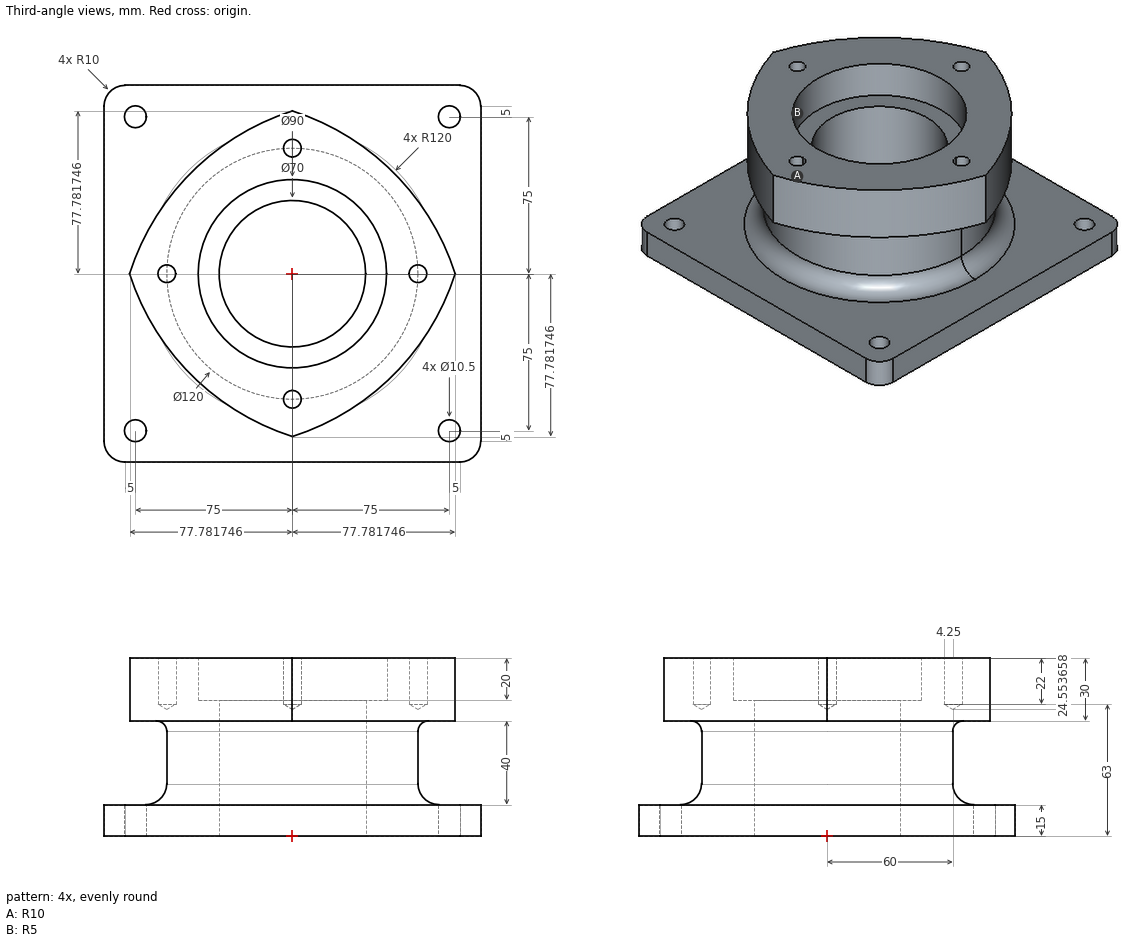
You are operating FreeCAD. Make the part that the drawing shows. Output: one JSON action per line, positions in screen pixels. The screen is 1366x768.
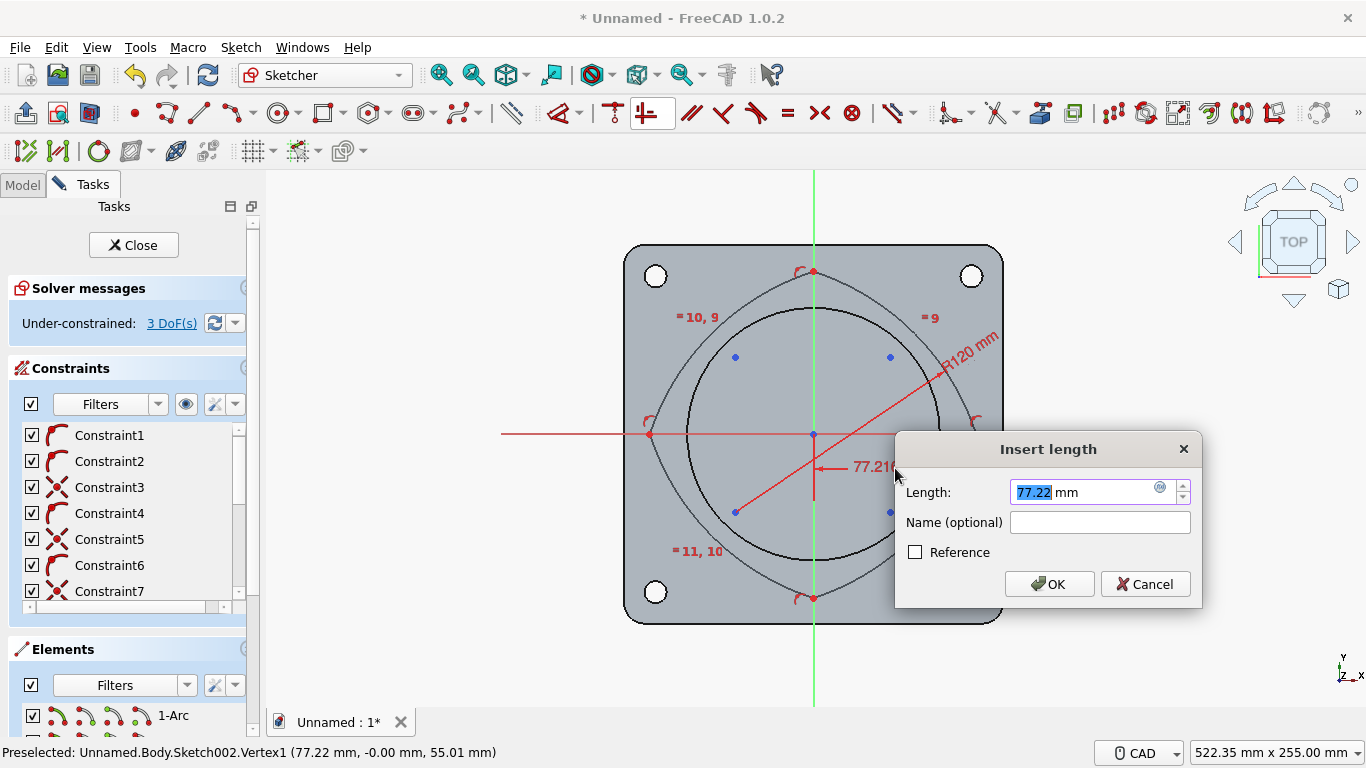
{"action": "type", "text": "77.781746"}
{"action": "key", "text": "Return"}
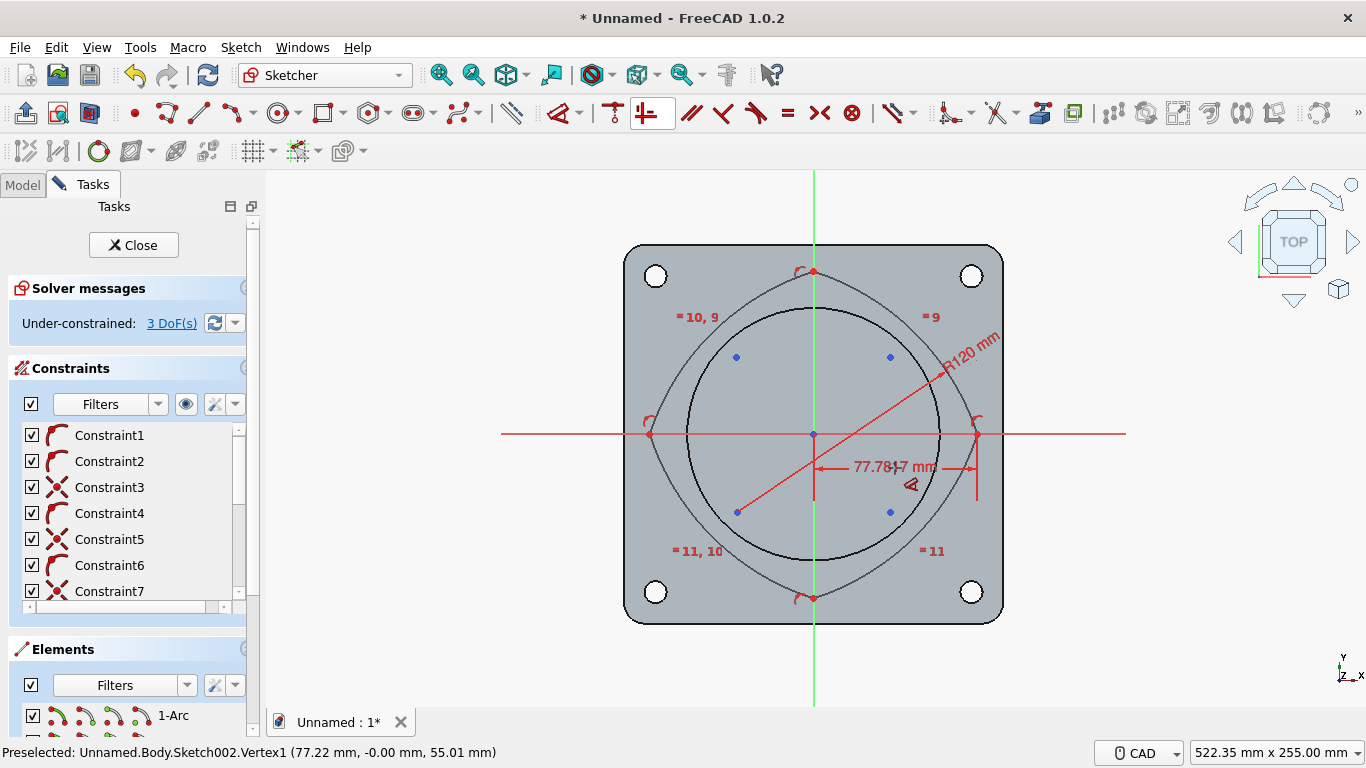
{"action": "left_click", "coordinate": [814, 272]}
{"action": "left_click", "coordinate": [848, 353]}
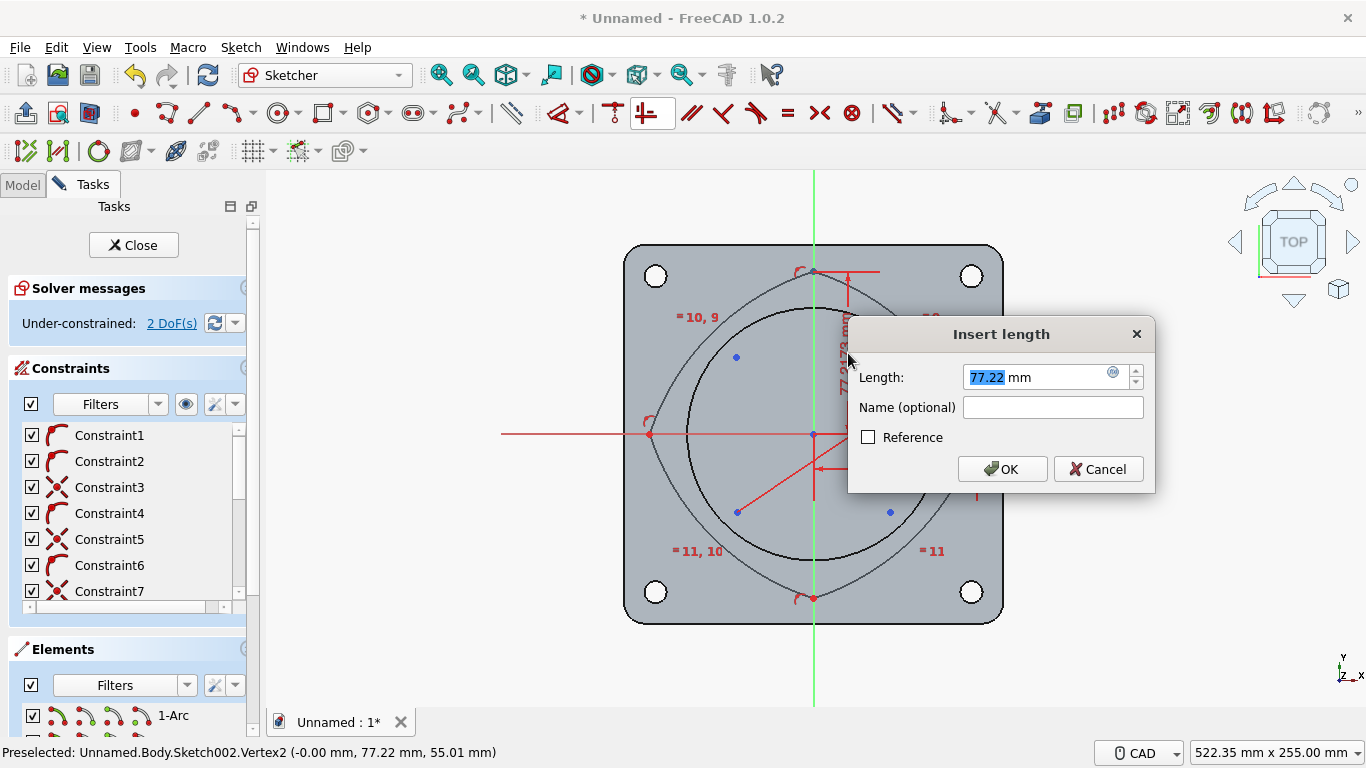
{"action": "type", "text": "77.781746"}
{"action": "key", "text": "Return"}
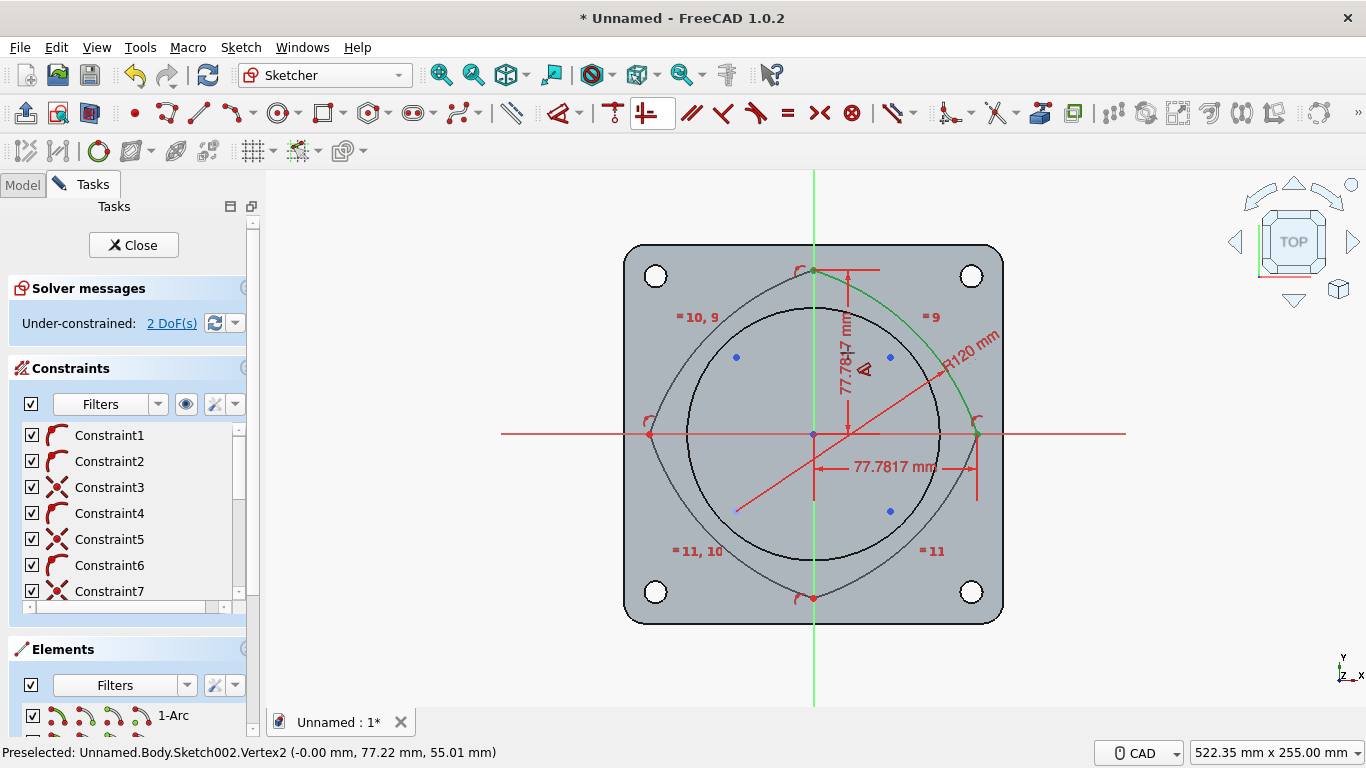
{"action": "left_click", "coordinate": [650, 434]}
{"action": "left_click", "coordinate": [732, 468]}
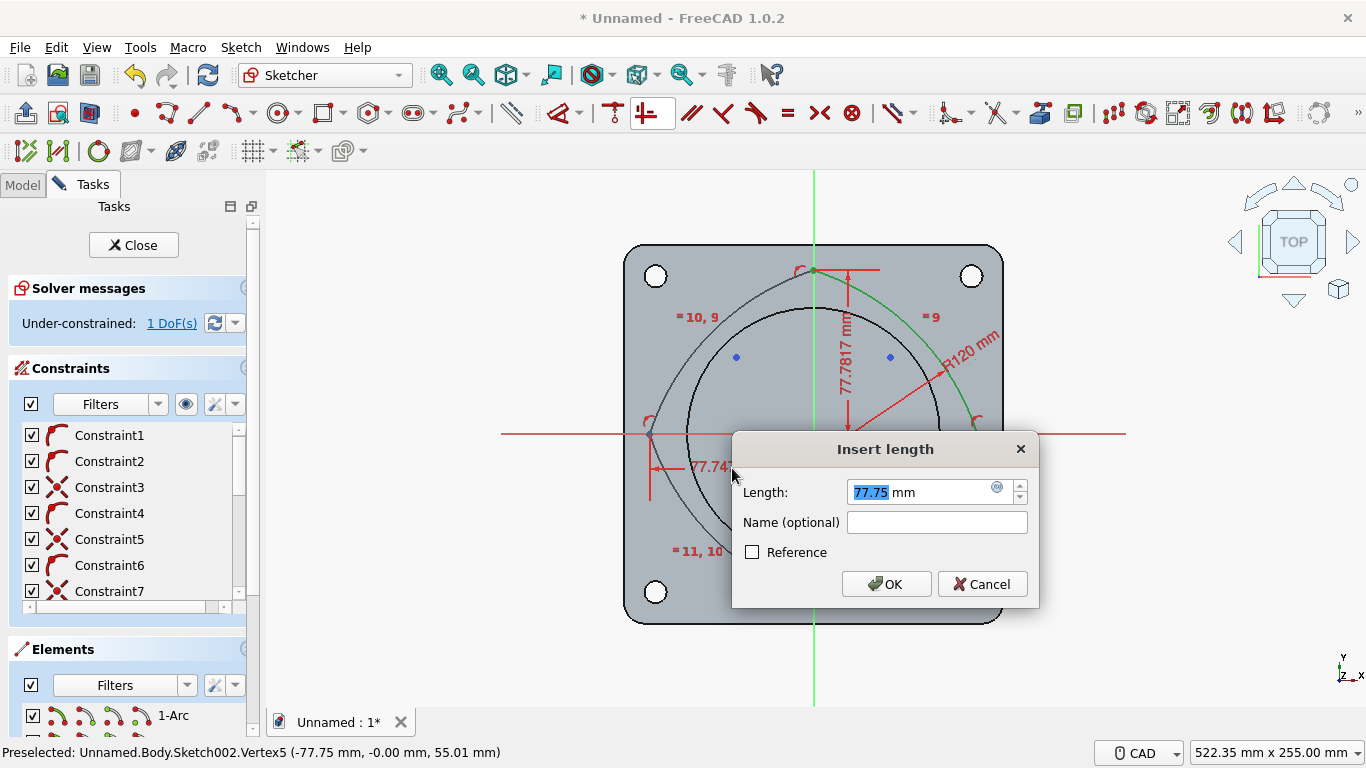
{"action": "type", "text": "77.781746"}
{"action": "key", "text": "Return"}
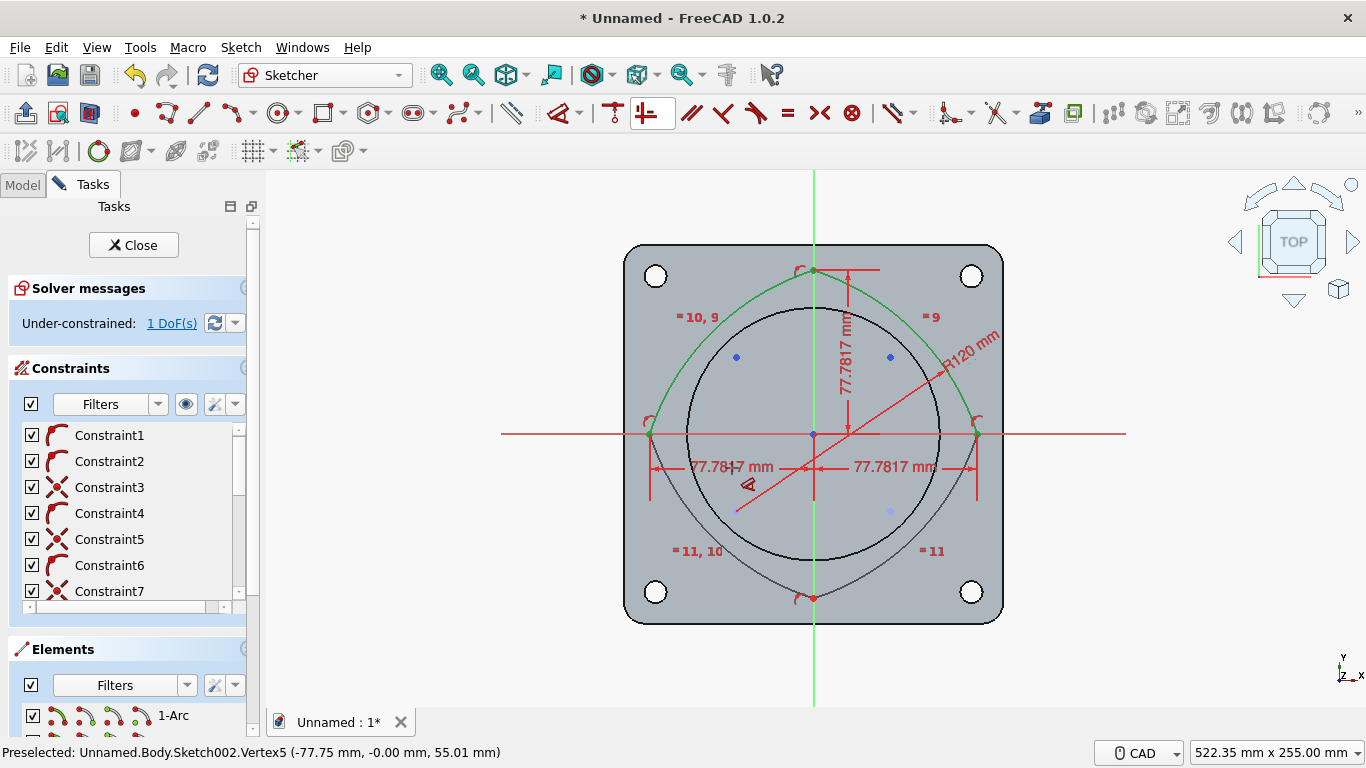
{"action": "left_click", "coordinate": [814, 598]}
{"action": "left_click", "coordinate": [848, 516]}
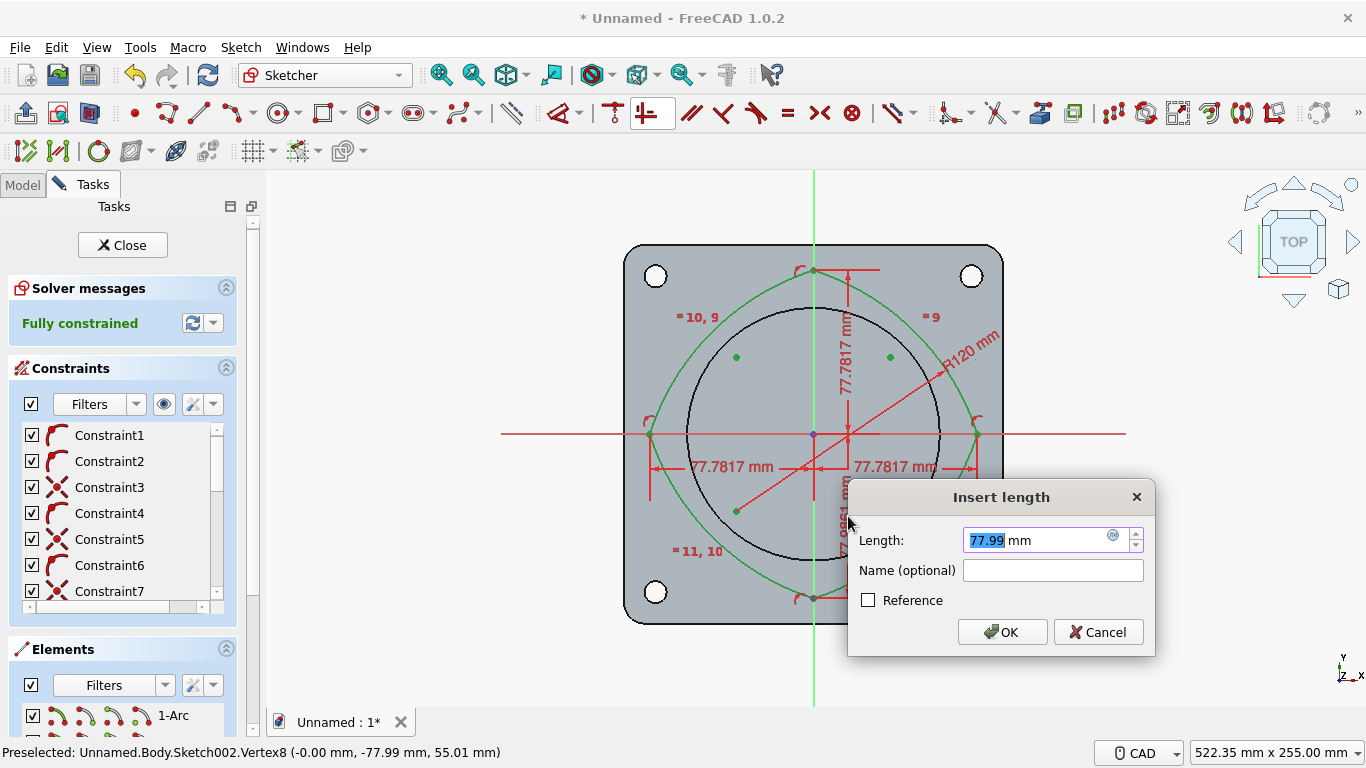
{"action": "type", "text": "77.781746"}
{"action": "key", "text": "Return"}
{"action": "key", "text": "Escape"}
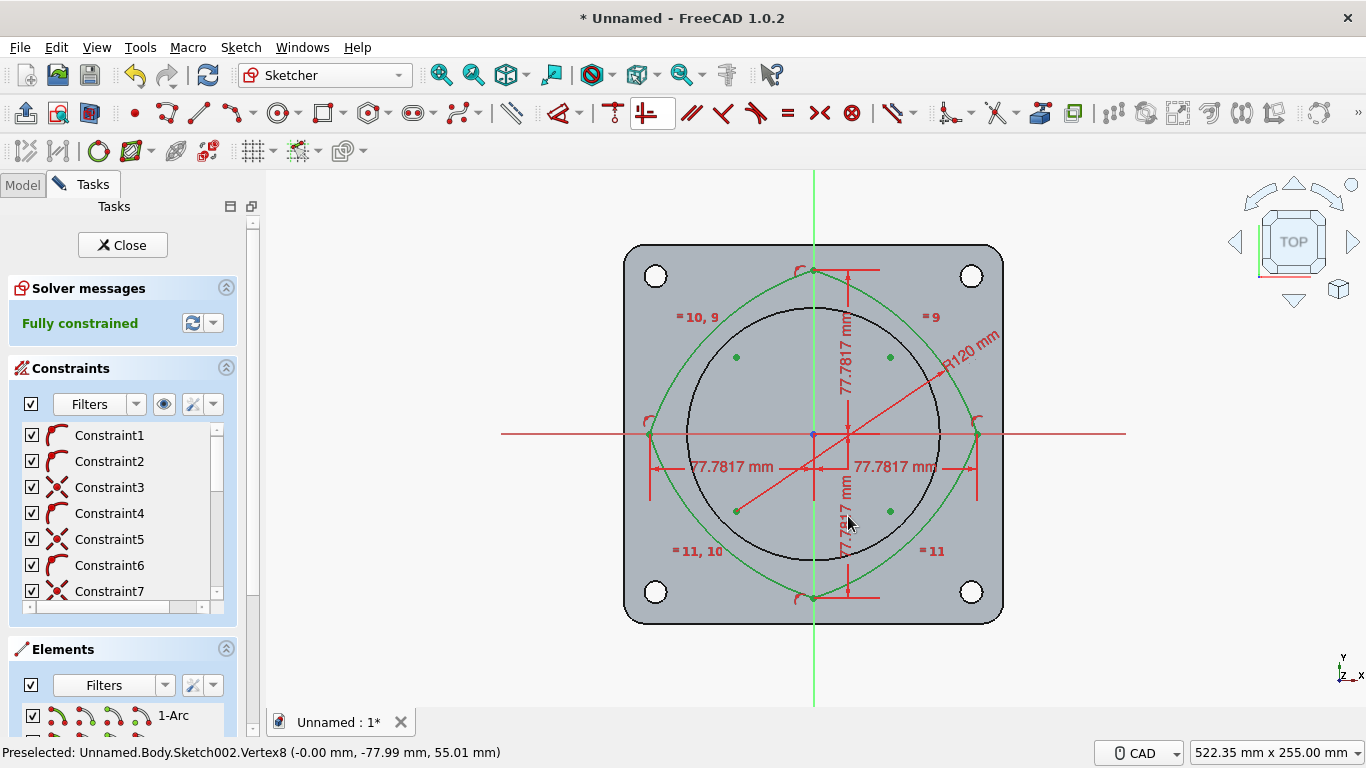
{"action": "left_click", "coordinate": [123, 245]}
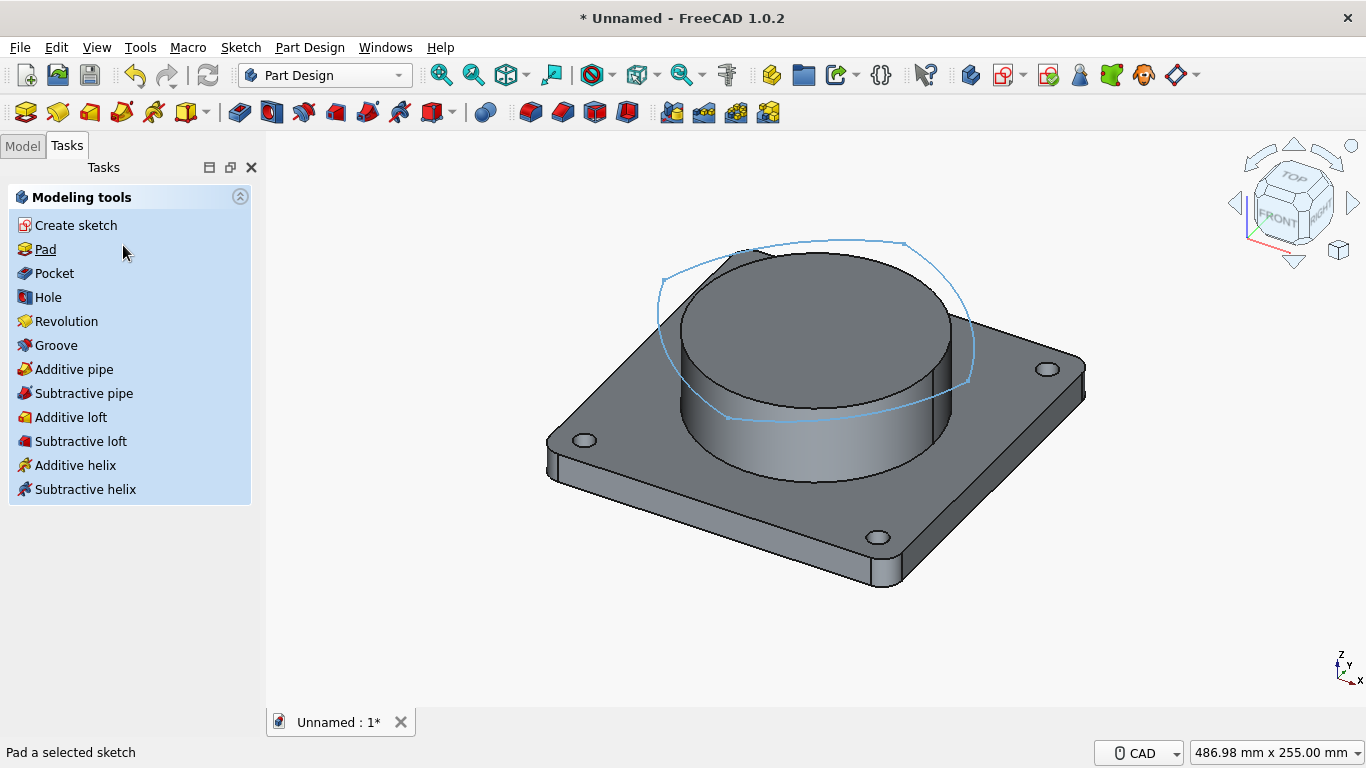
{"action": "left_click", "coordinate": [26, 112]}